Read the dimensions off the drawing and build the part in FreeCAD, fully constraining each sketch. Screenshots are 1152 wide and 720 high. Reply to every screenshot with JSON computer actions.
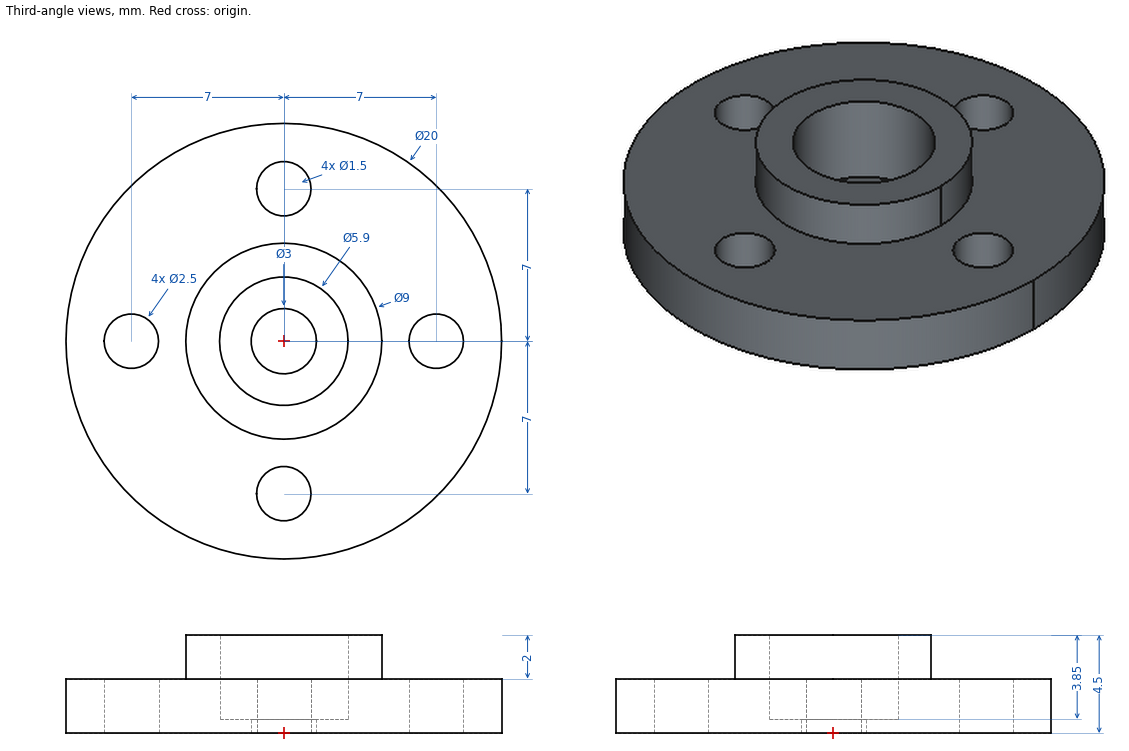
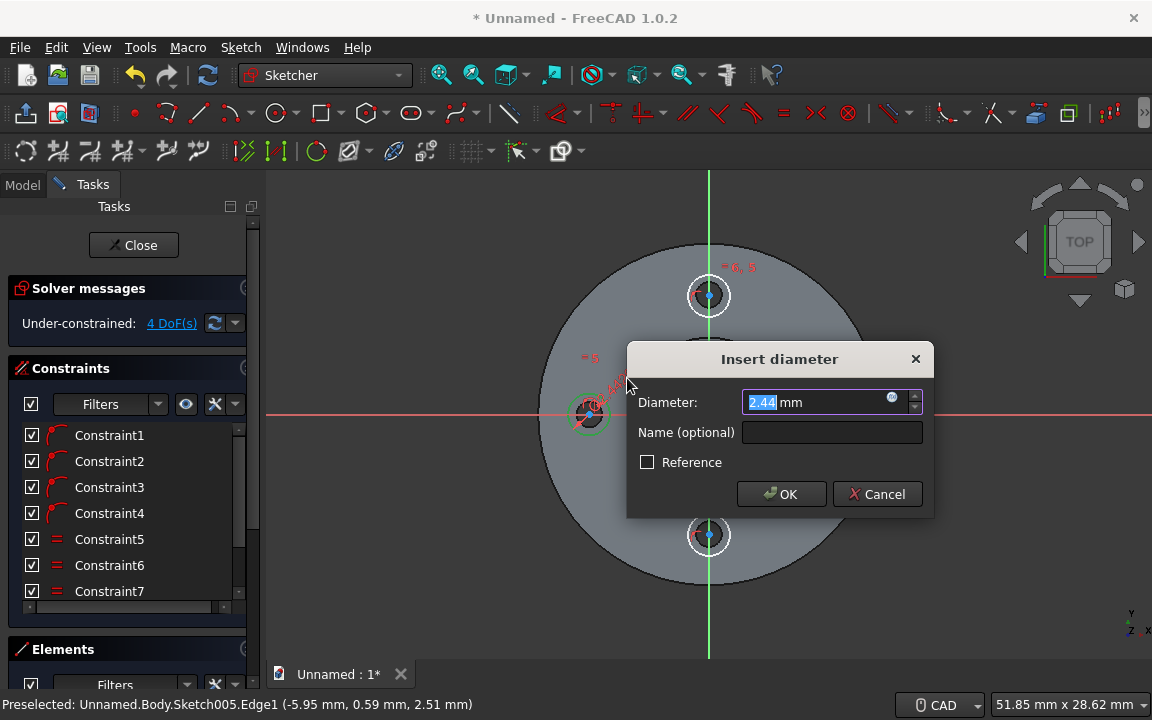
{"action": "type", "text": "2.5"}
{"action": "key", "text": "Return"}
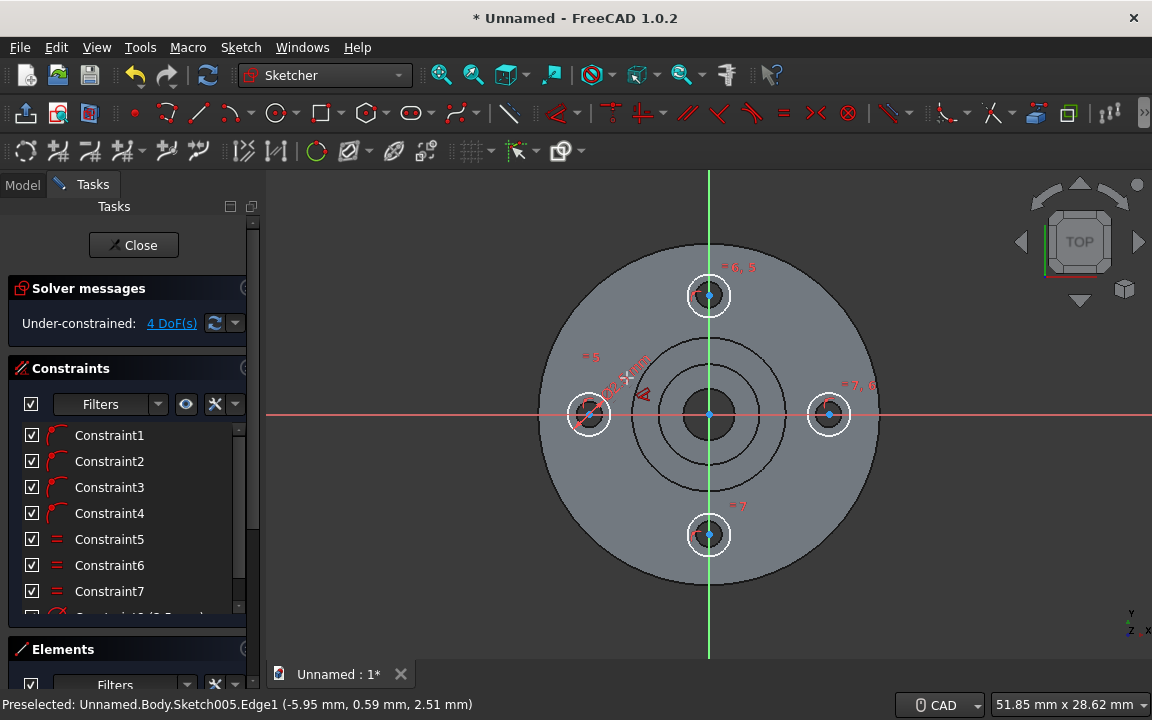
{"action": "left_click", "coordinate": [589, 414]}
{"action": "left_click", "coordinate": [649, 448]}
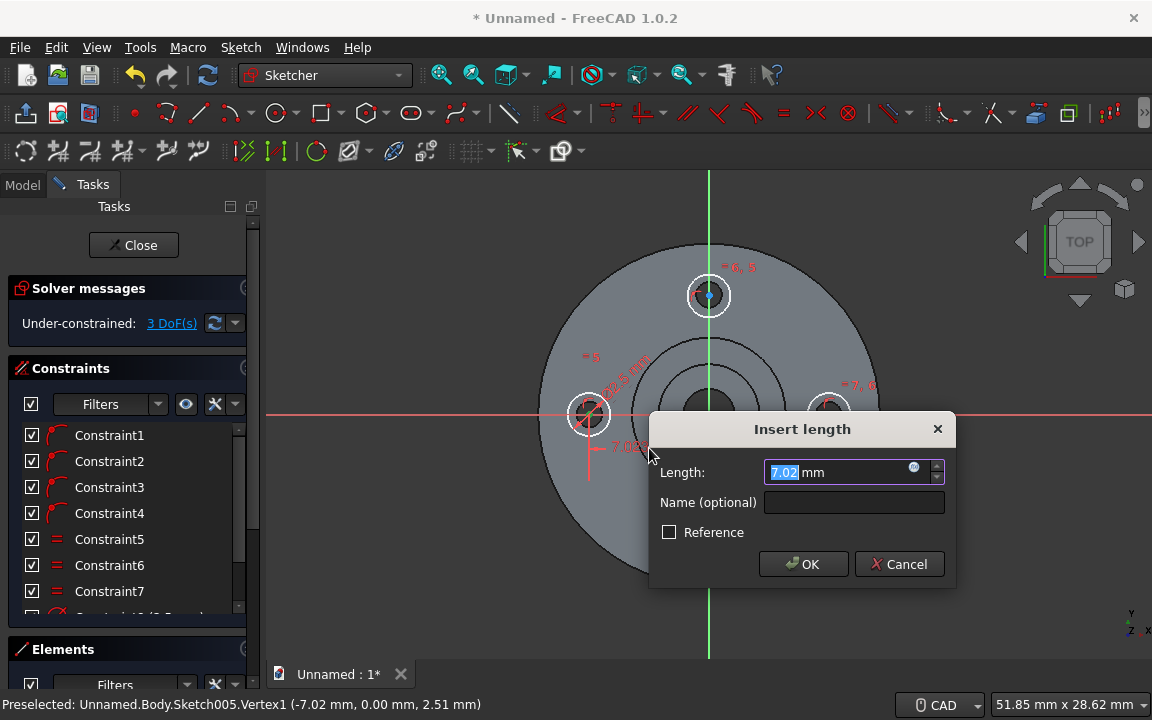
{"action": "type", "text": "7"}
{"action": "key", "text": "Return"}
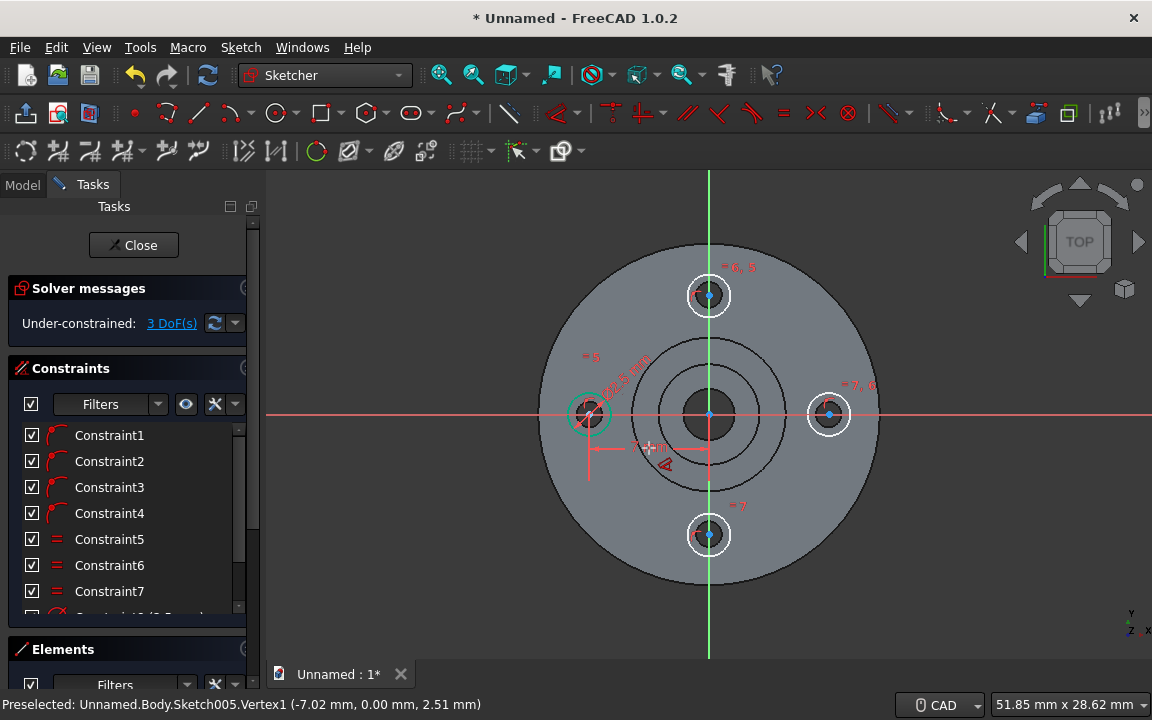
{"action": "left_click", "coordinate": [709, 296]}
{"action": "left_click", "coordinate": [743, 355]}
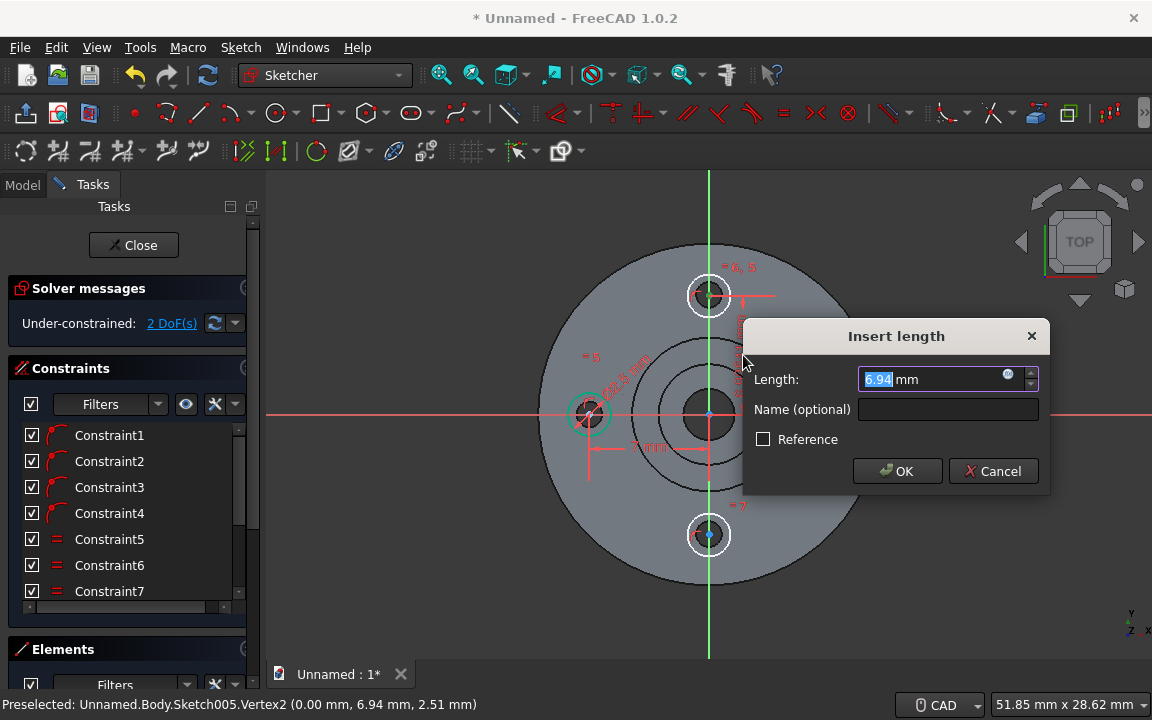
{"action": "type", "text": "7"}
{"action": "key", "text": "Return"}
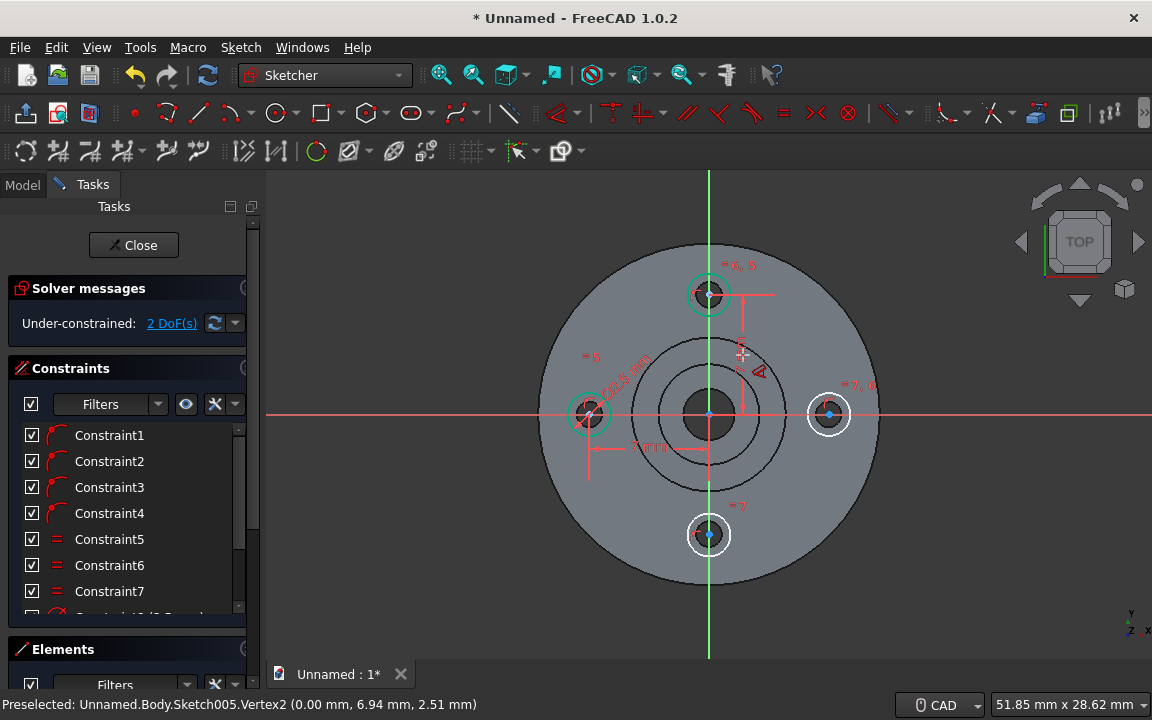
{"action": "left_click", "coordinate": [829, 414]}
{"action": "left_click", "coordinate": [769, 448]}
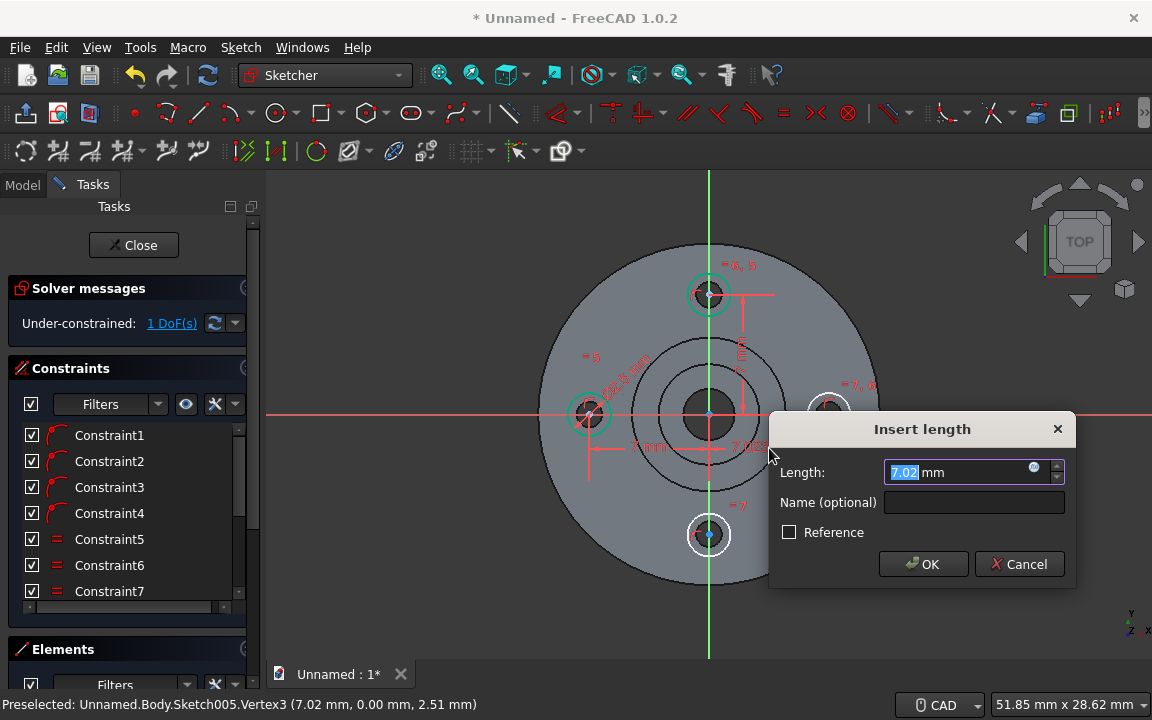
{"action": "type", "text": "7"}
{"action": "key", "text": "Return"}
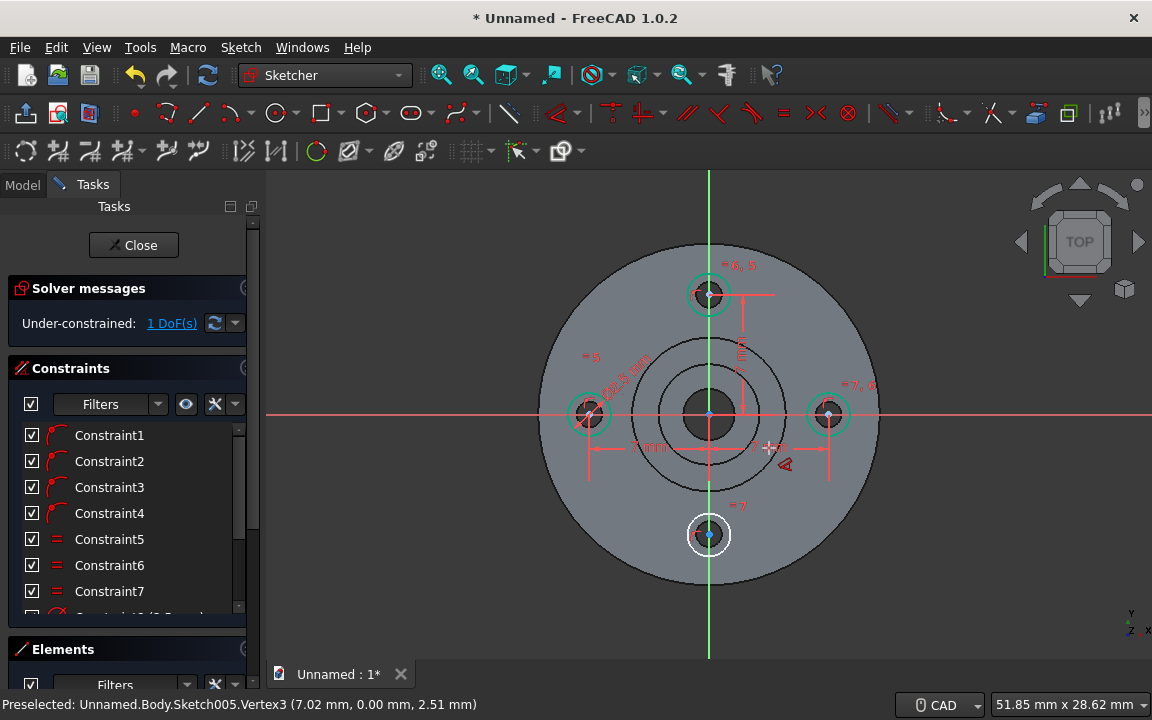
{"action": "left_click", "coordinate": [709, 535]}
{"action": "left_click", "coordinate": [743, 475]}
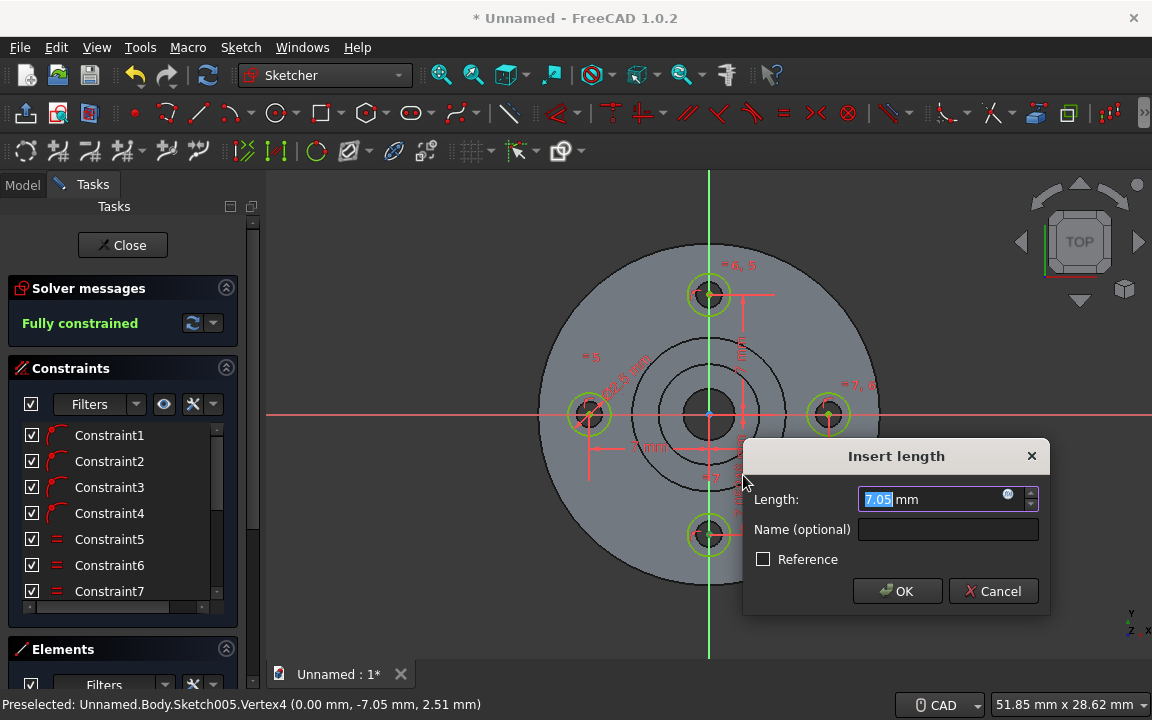
{"action": "type", "text": "7"}
{"action": "key", "text": "Return"}
{"action": "key", "text": "Escape"}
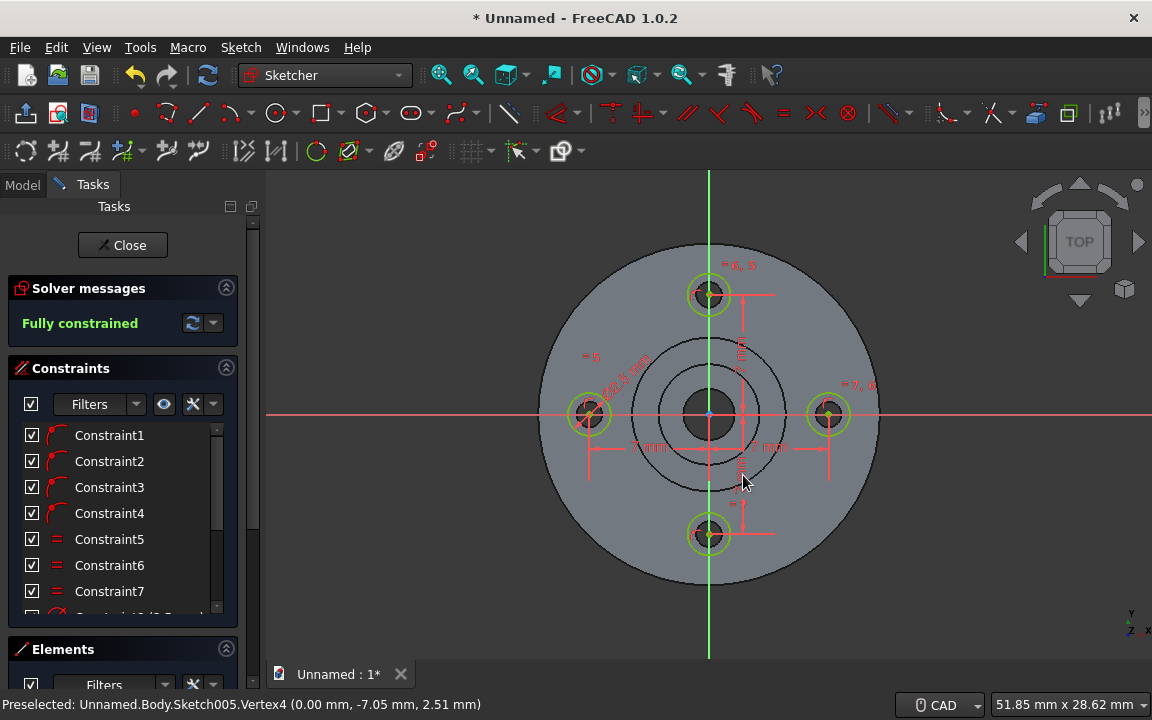
{"action": "left_click", "coordinate": [123, 245]}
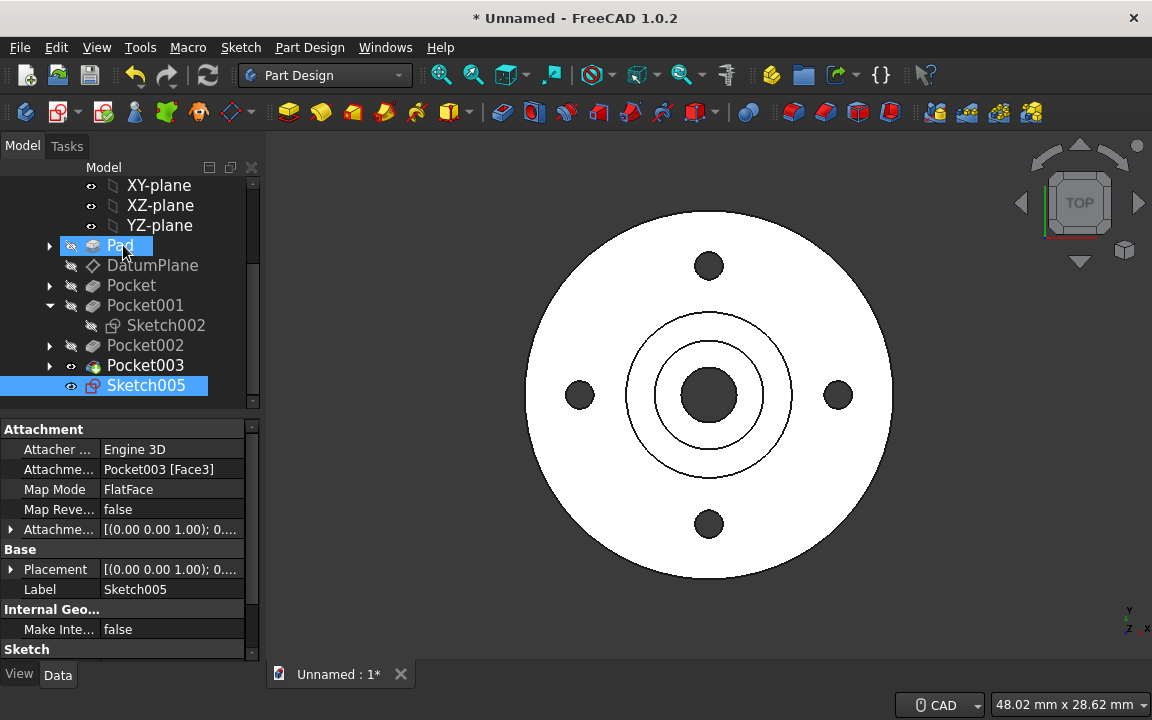
{"action": "left_click", "coordinate": [504, 112]}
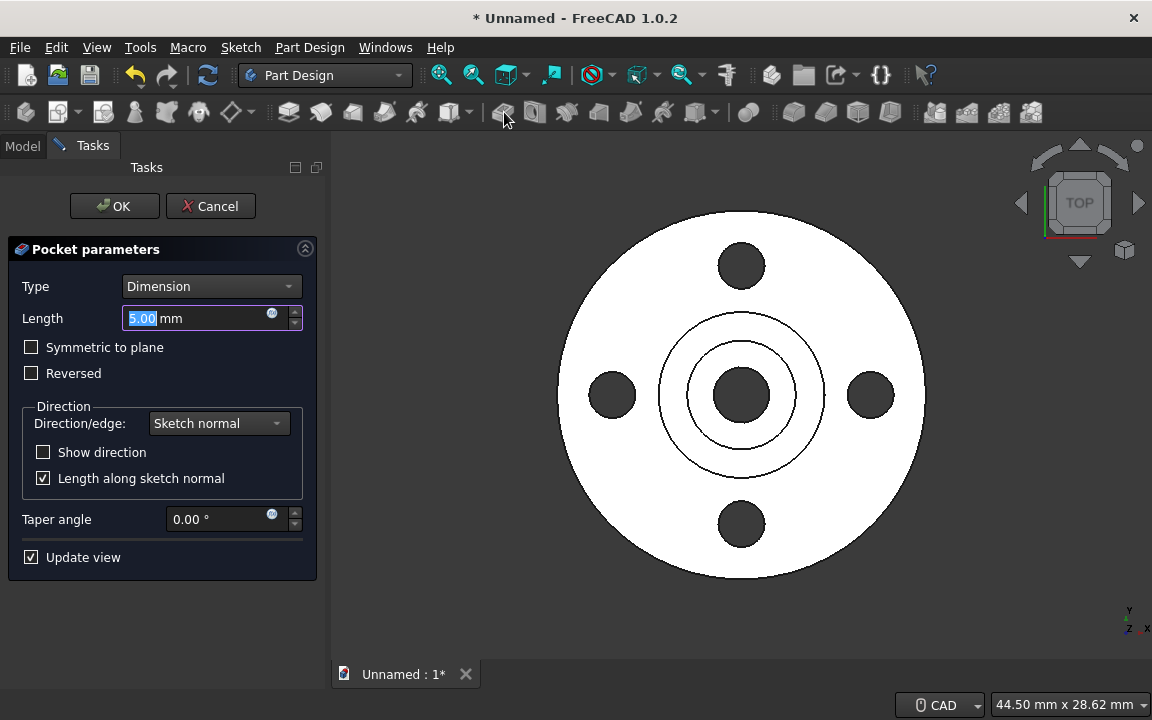
{"action": "left_click", "coordinate": [212, 286]}